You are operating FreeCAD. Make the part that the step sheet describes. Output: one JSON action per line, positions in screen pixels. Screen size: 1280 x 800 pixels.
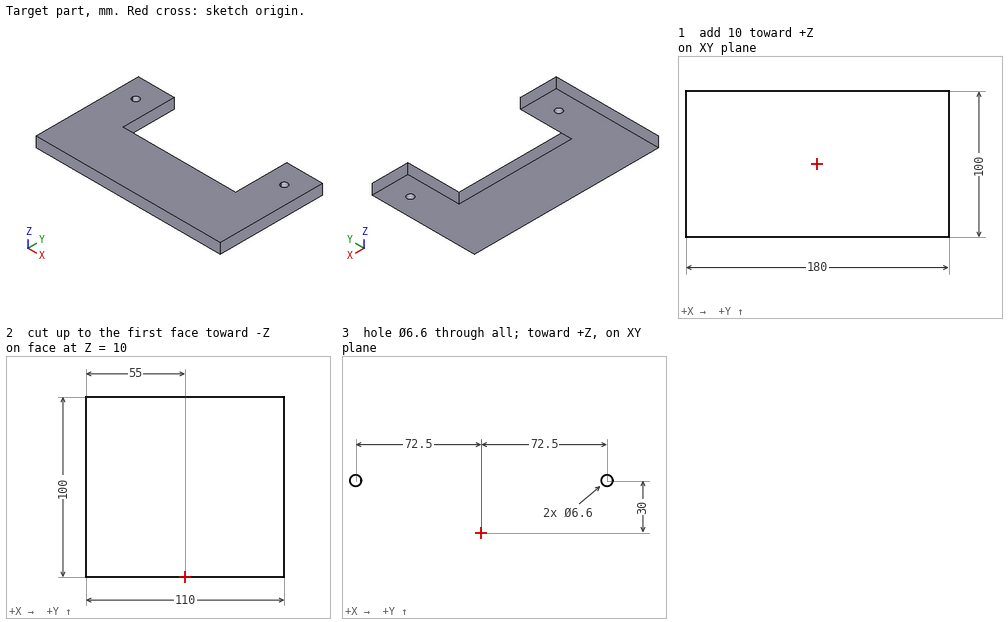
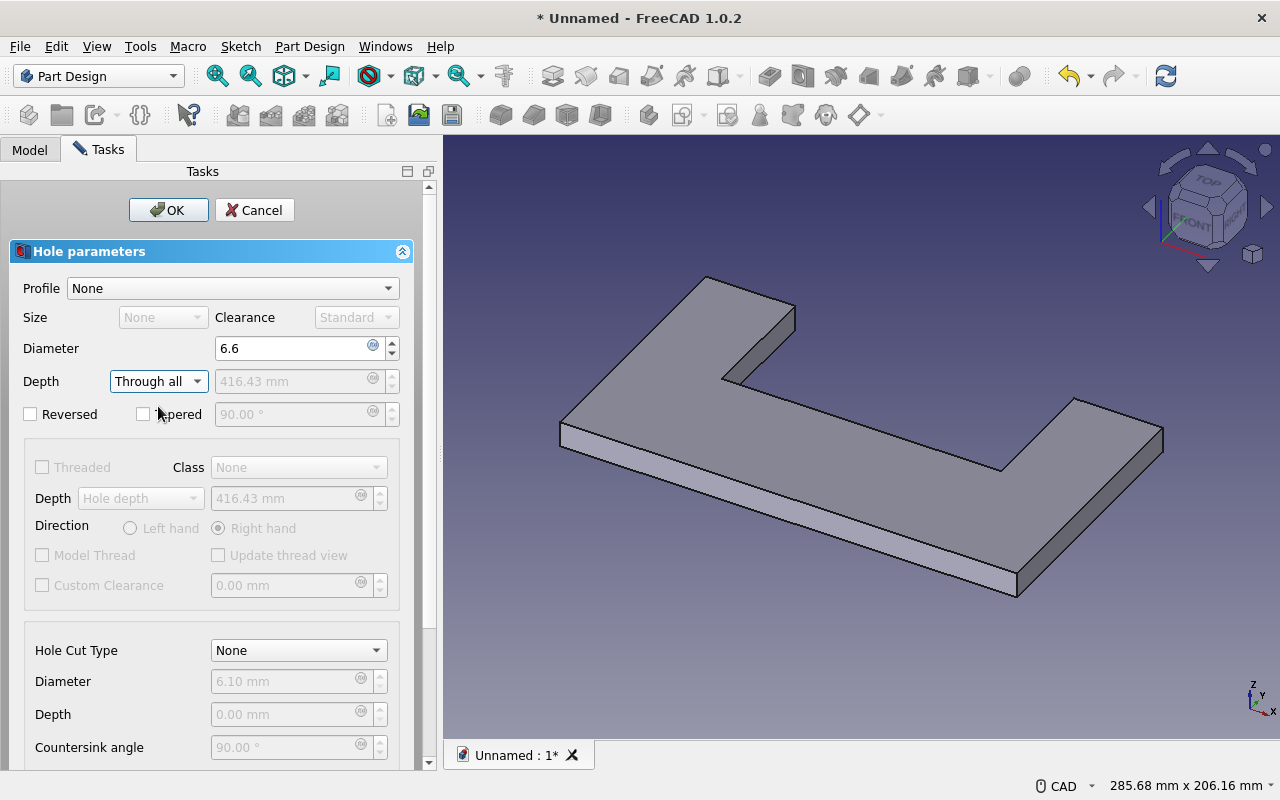
{"action": "left_click", "coordinate": [31, 414]}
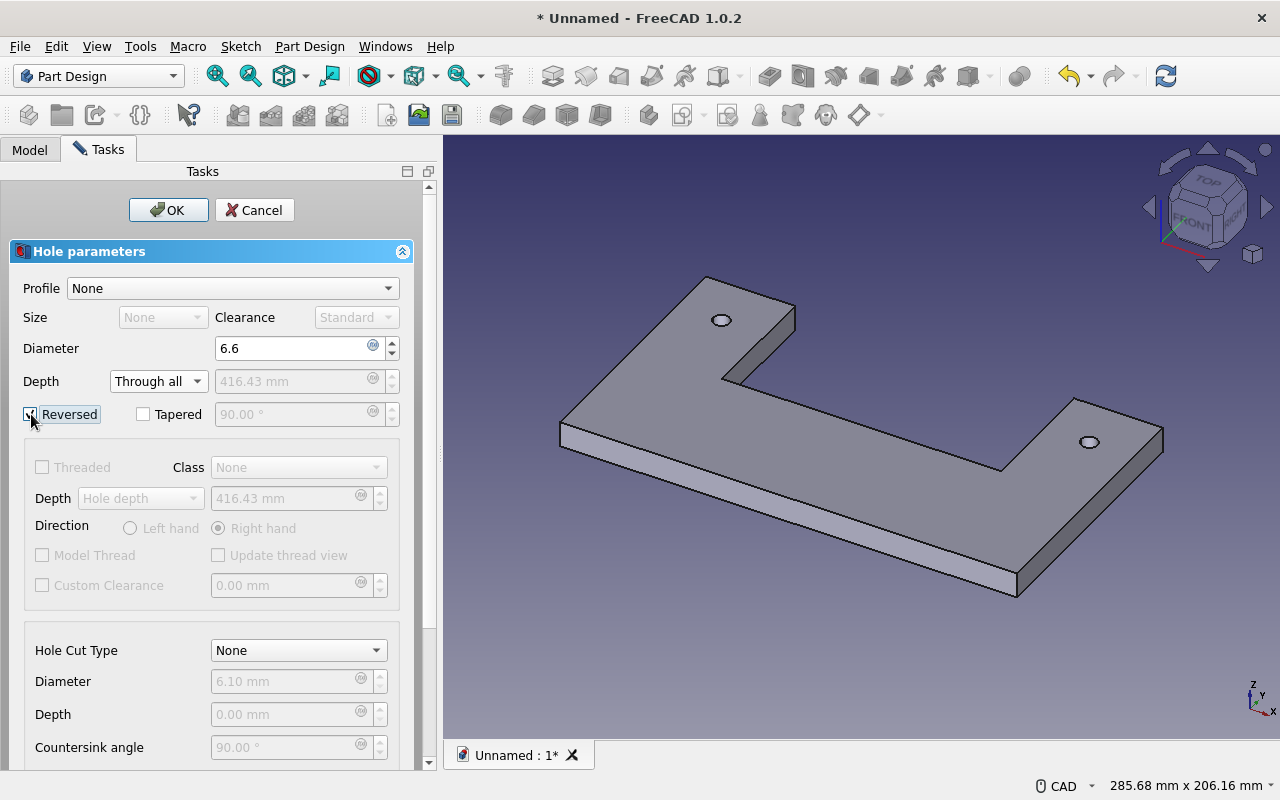
{"action": "left_click", "coordinate": [169, 210]}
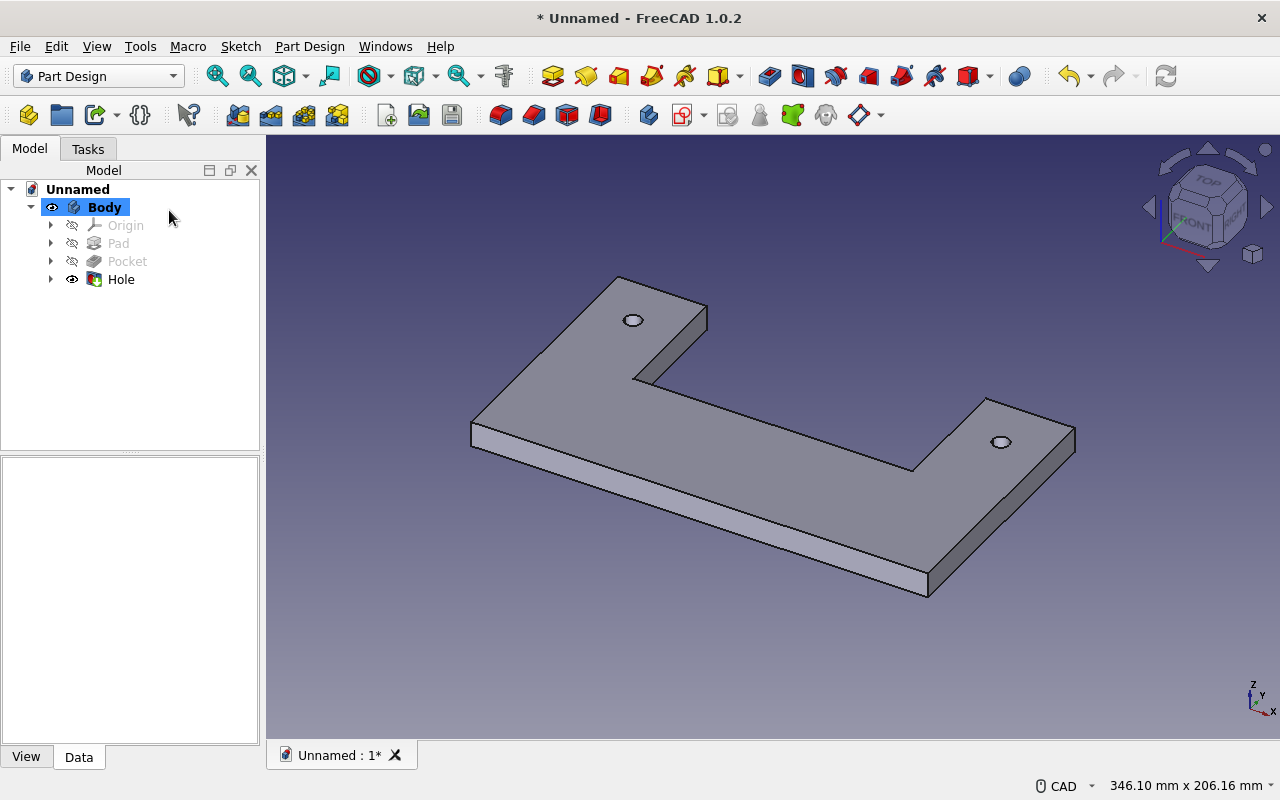
{"action": "key", "text": "0"}